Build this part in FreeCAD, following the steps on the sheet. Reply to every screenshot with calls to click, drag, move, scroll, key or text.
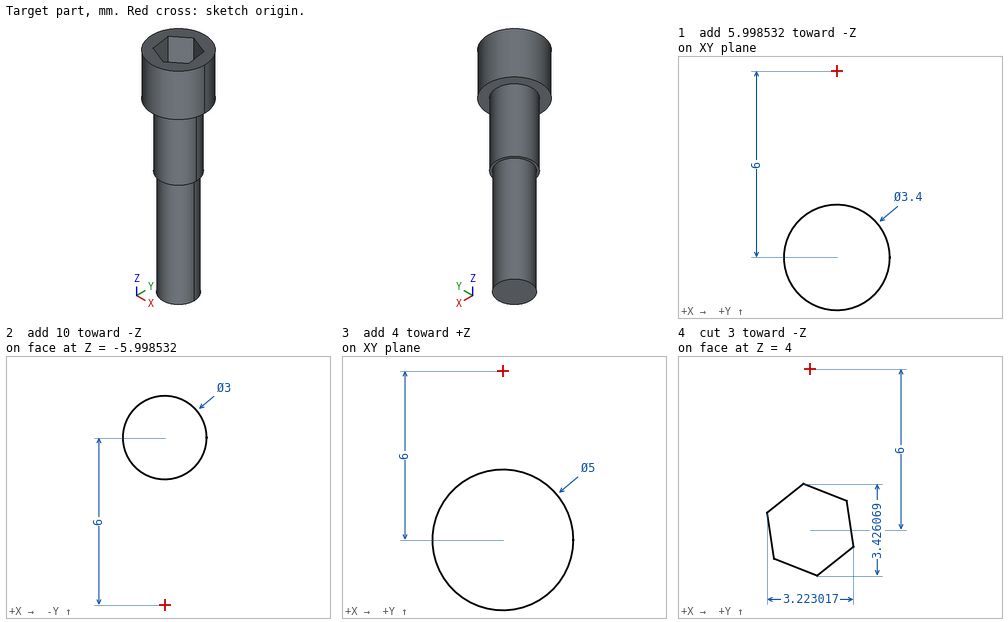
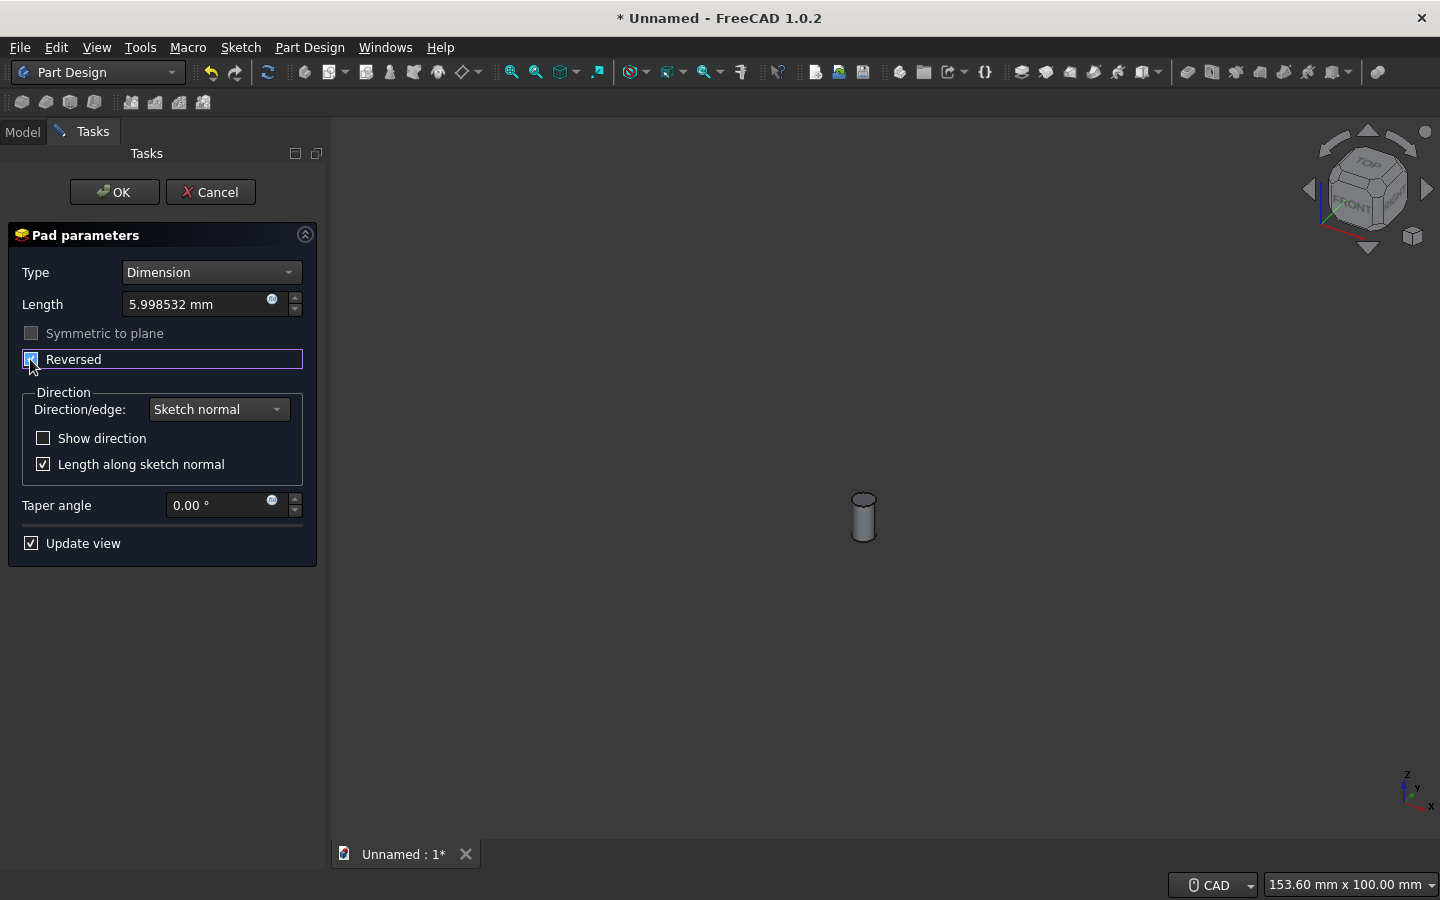
click(115, 192)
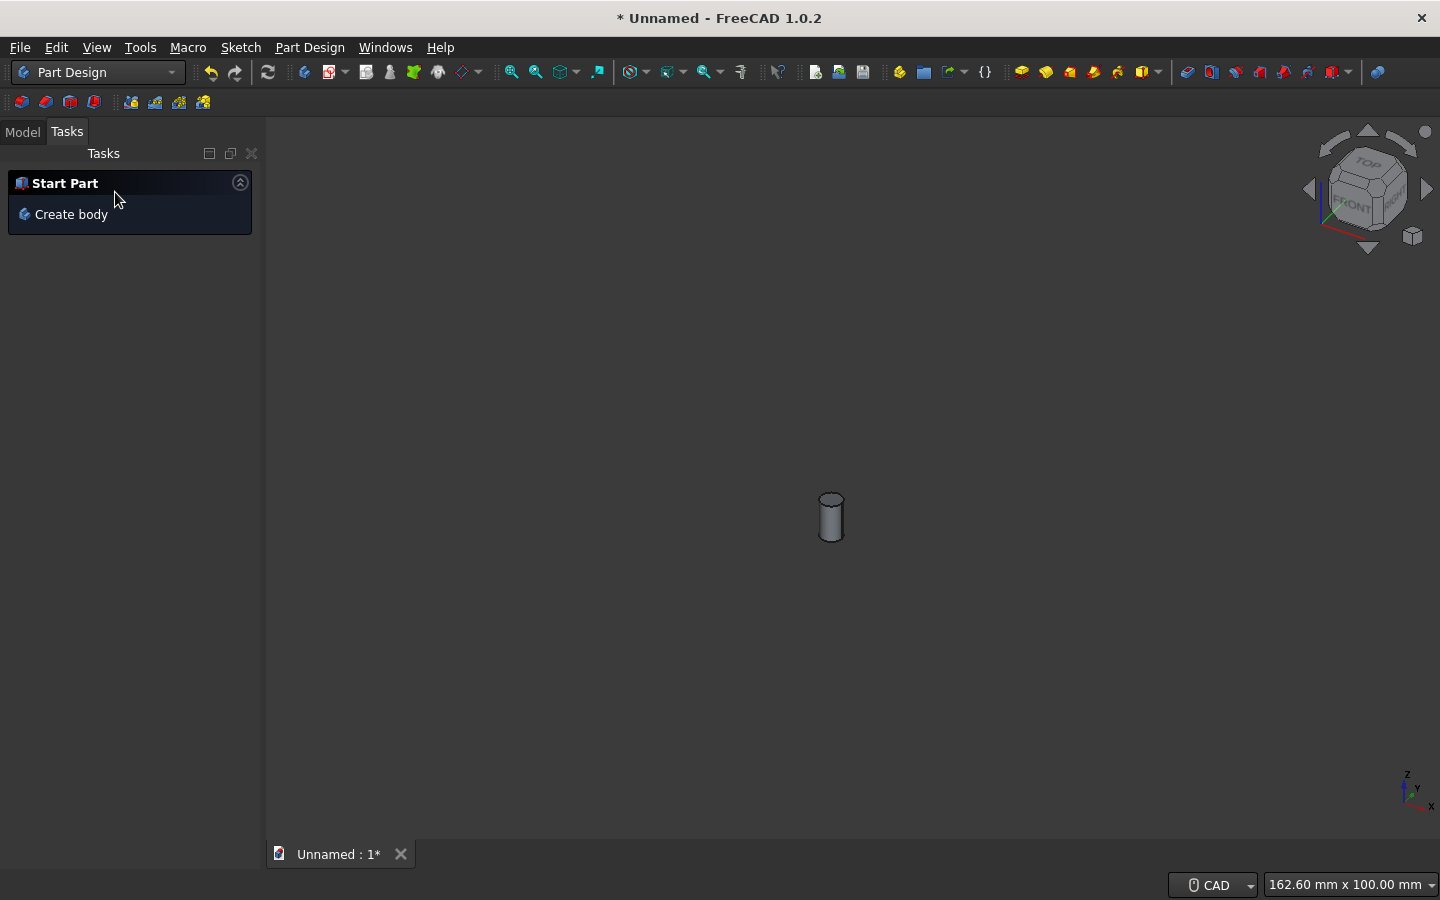
key(v)
key(f)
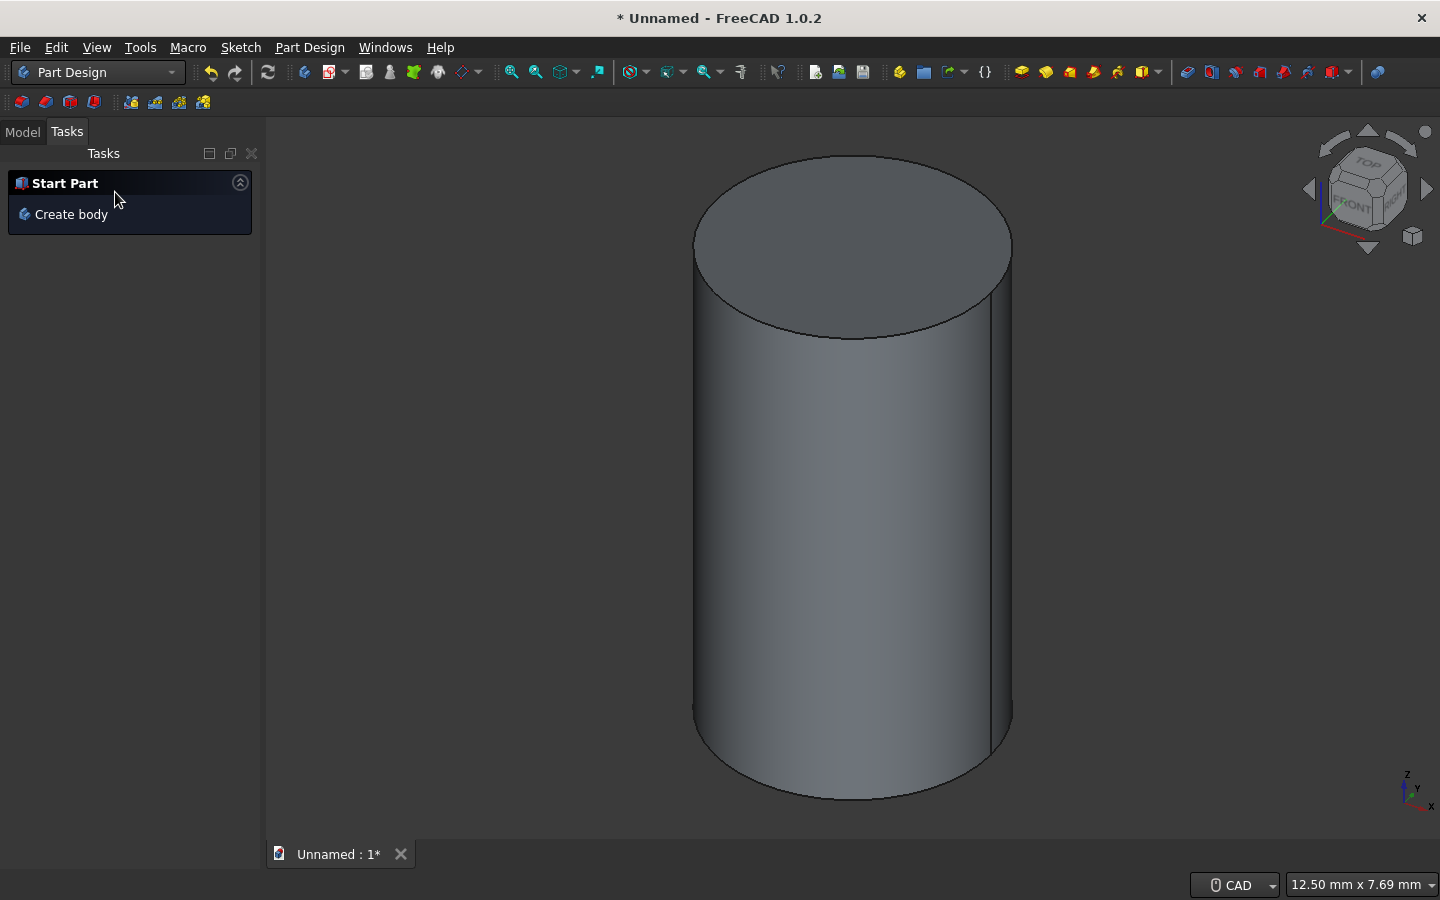
key(5)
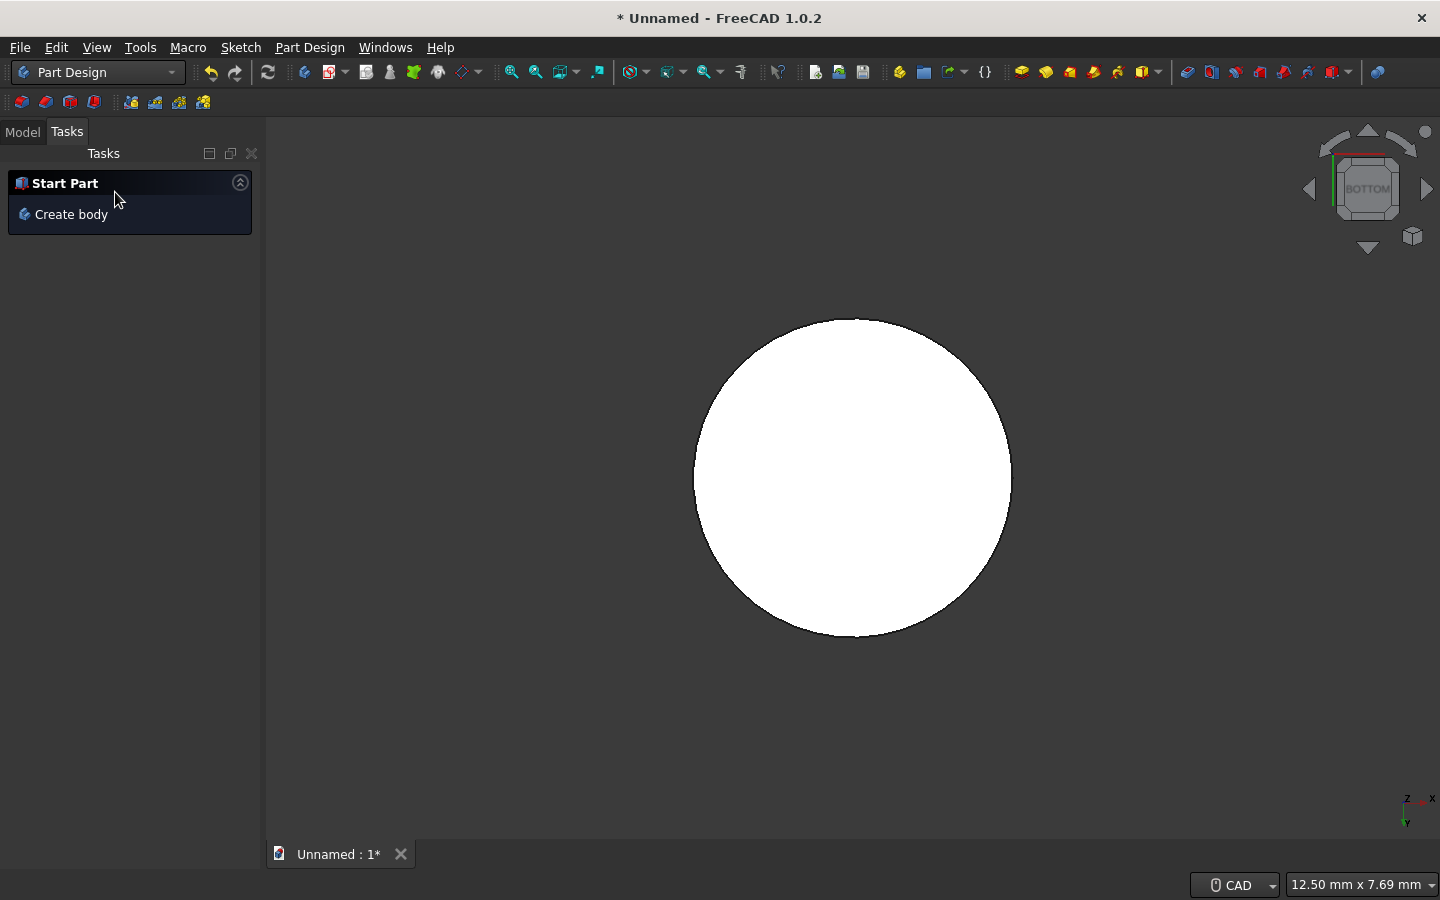
key(v)
key(f)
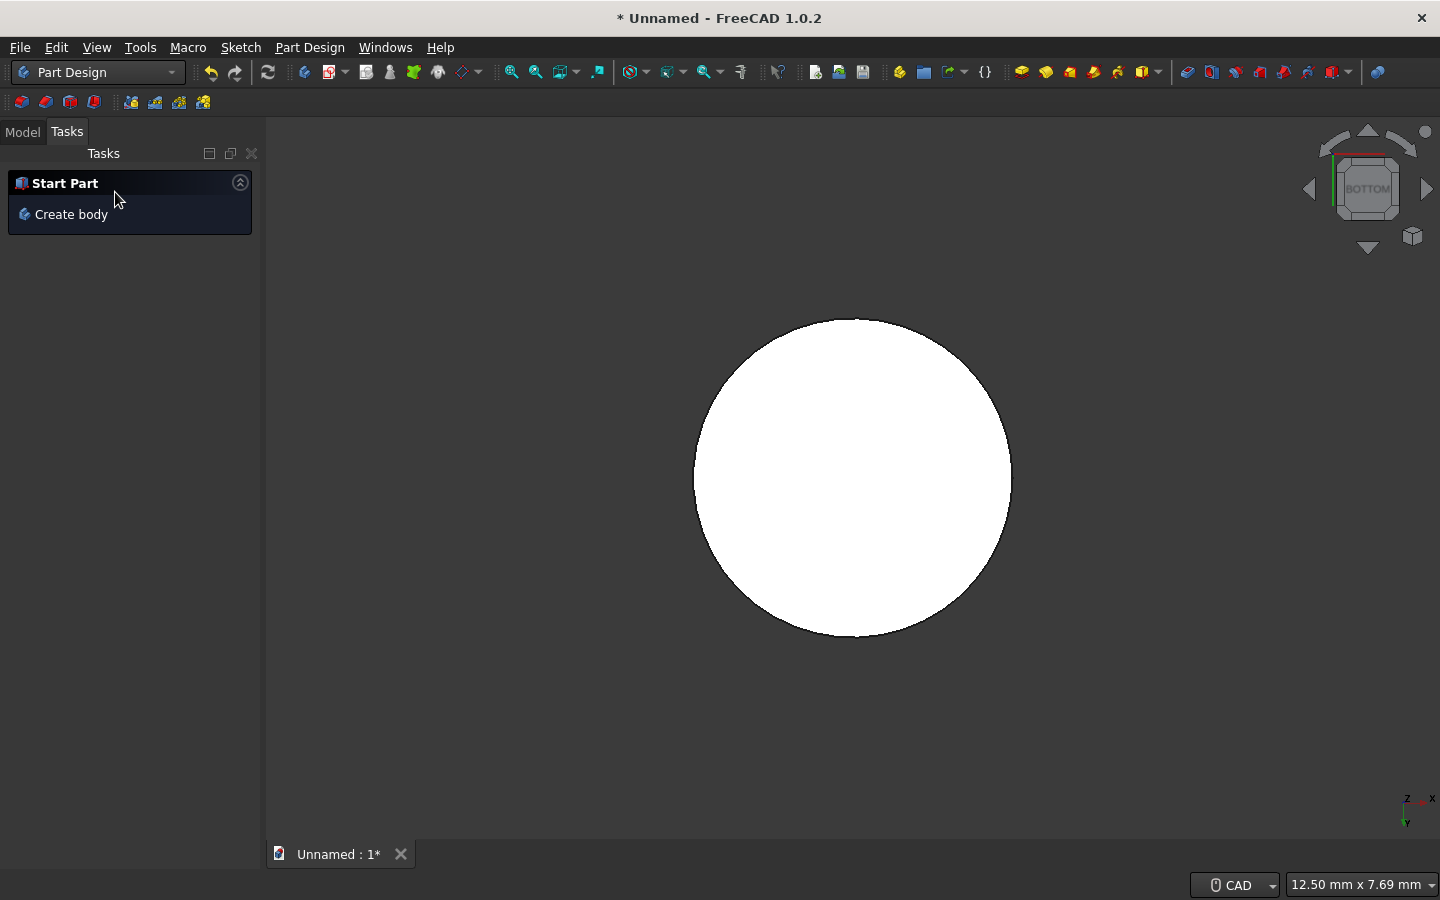
click(853, 477)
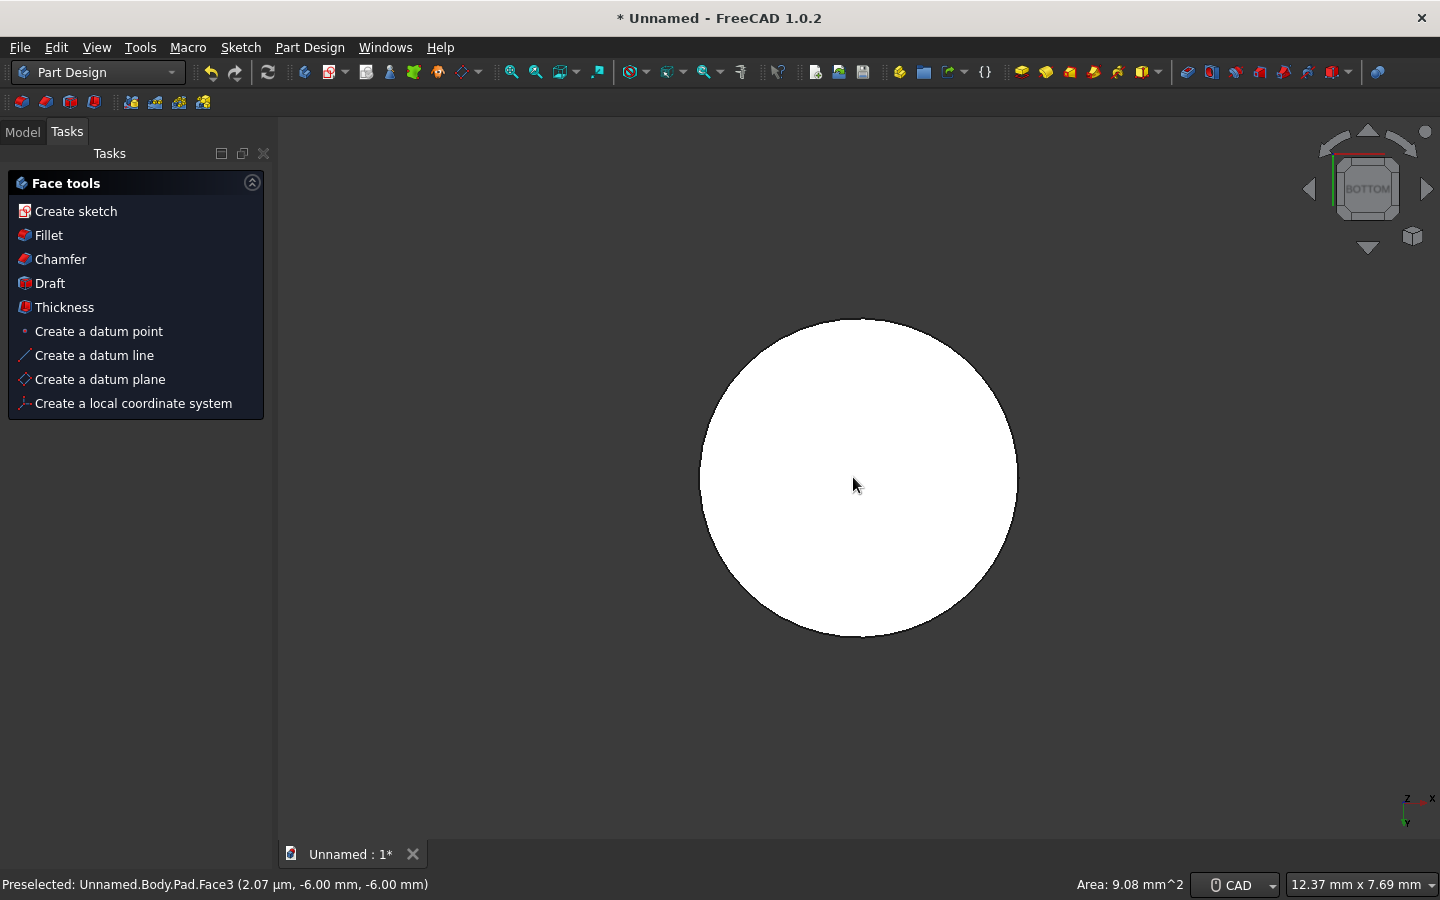
click(330, 72)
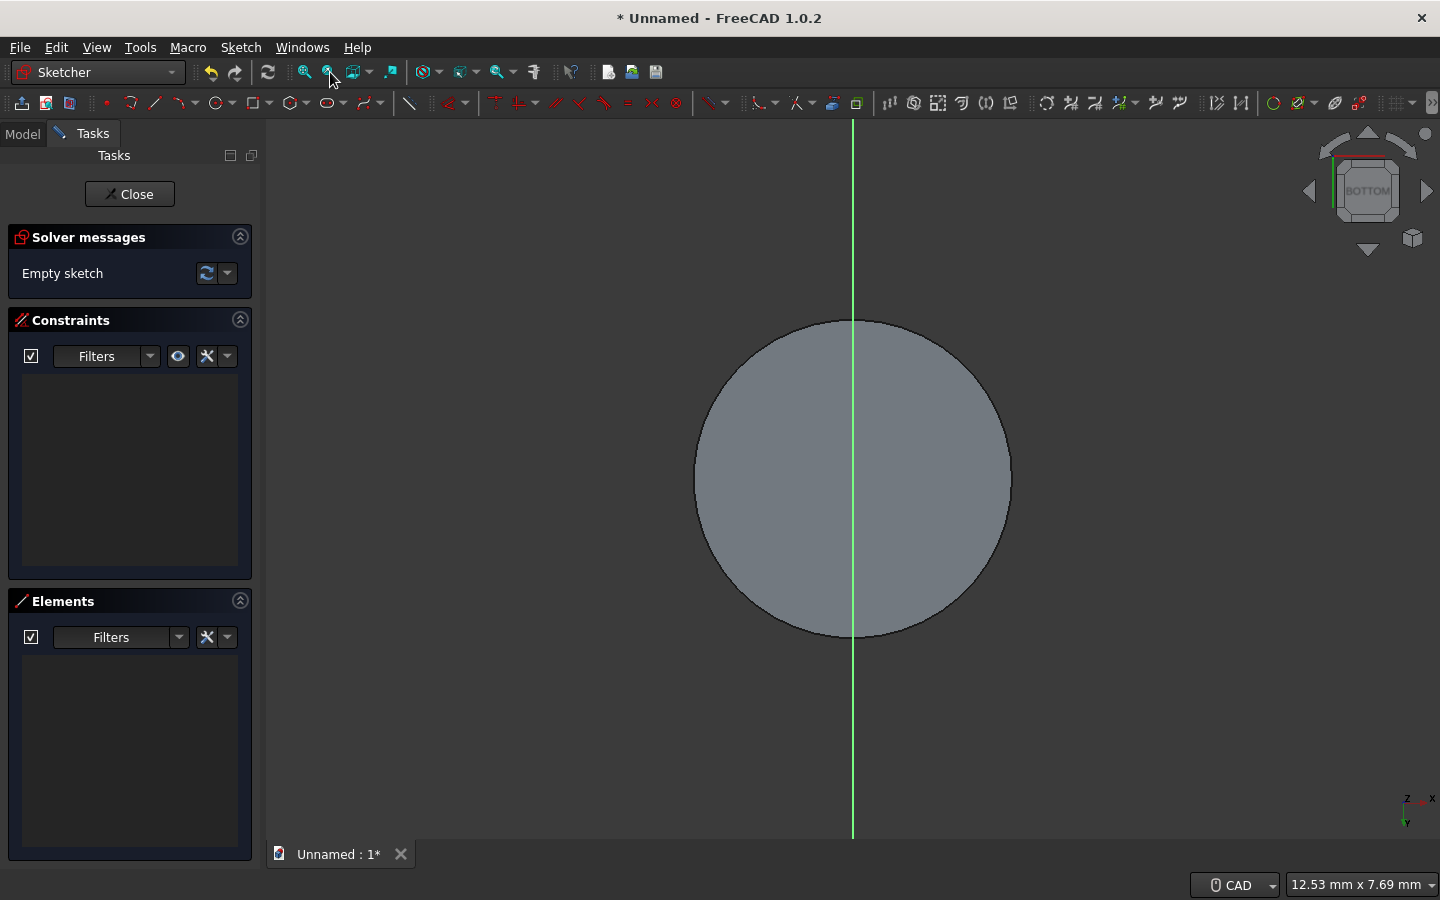
scroll(936, 479, up, 3)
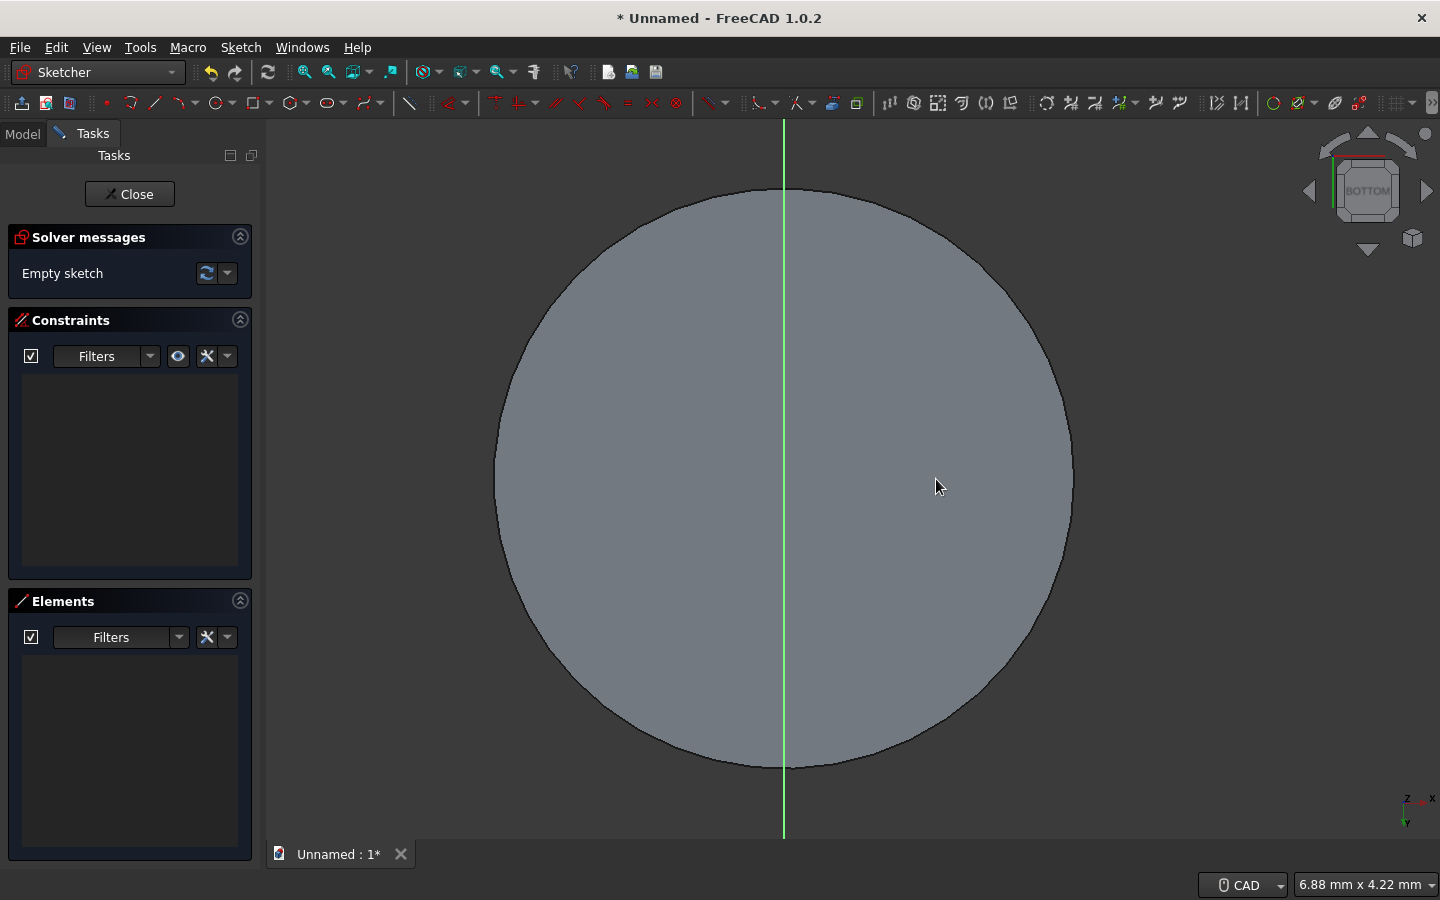
key(g)
key(c)